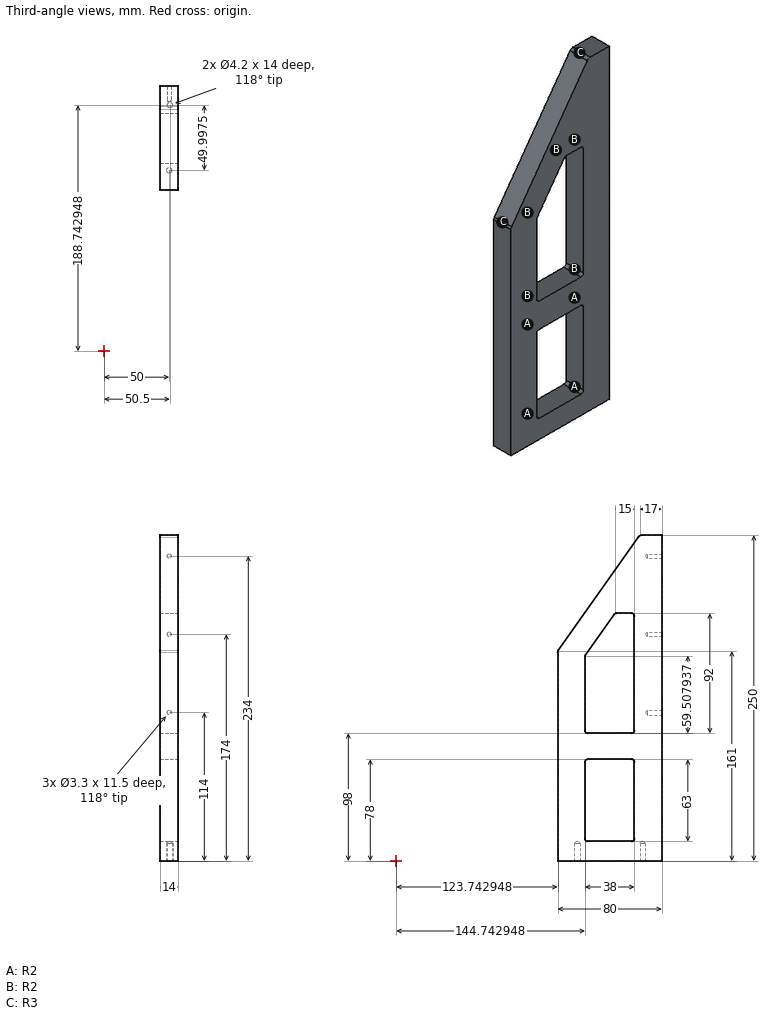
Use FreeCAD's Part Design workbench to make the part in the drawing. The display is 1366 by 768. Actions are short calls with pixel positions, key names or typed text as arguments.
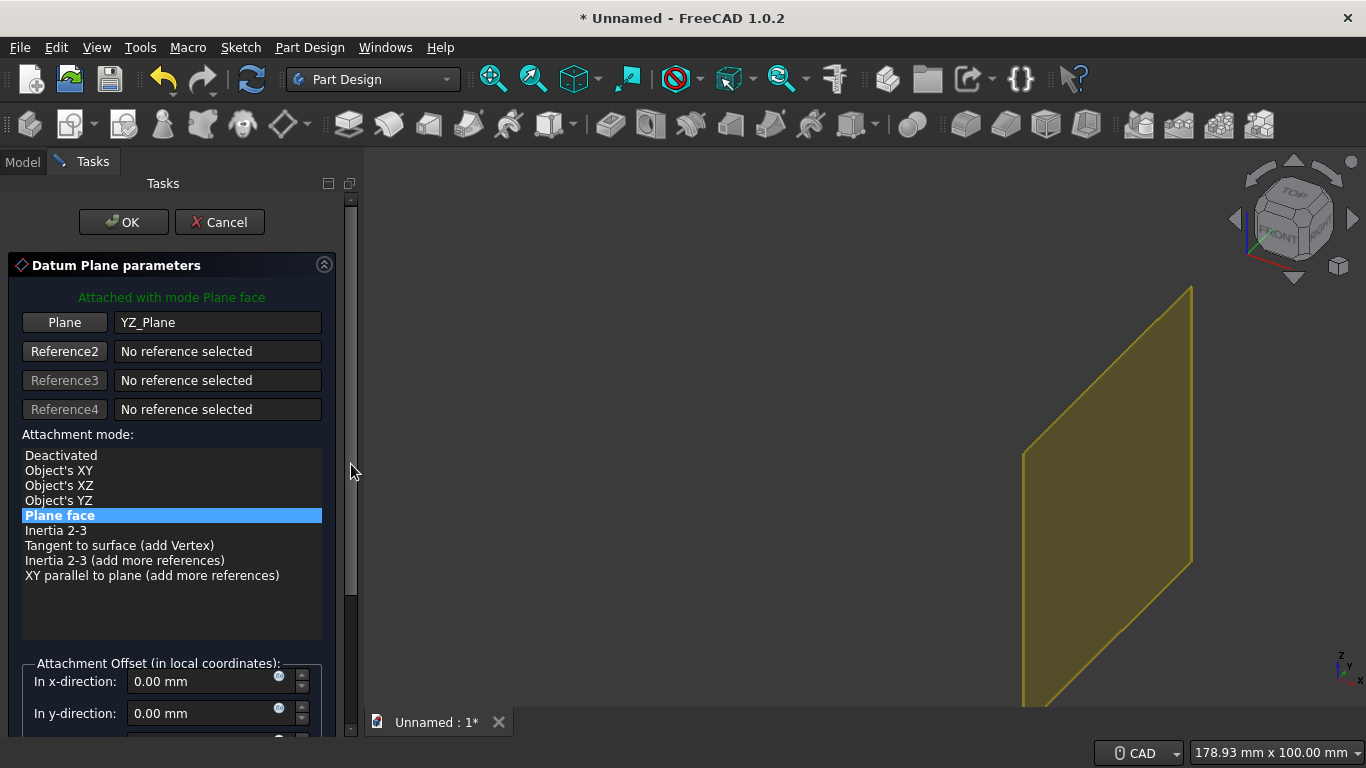
click(124, 222)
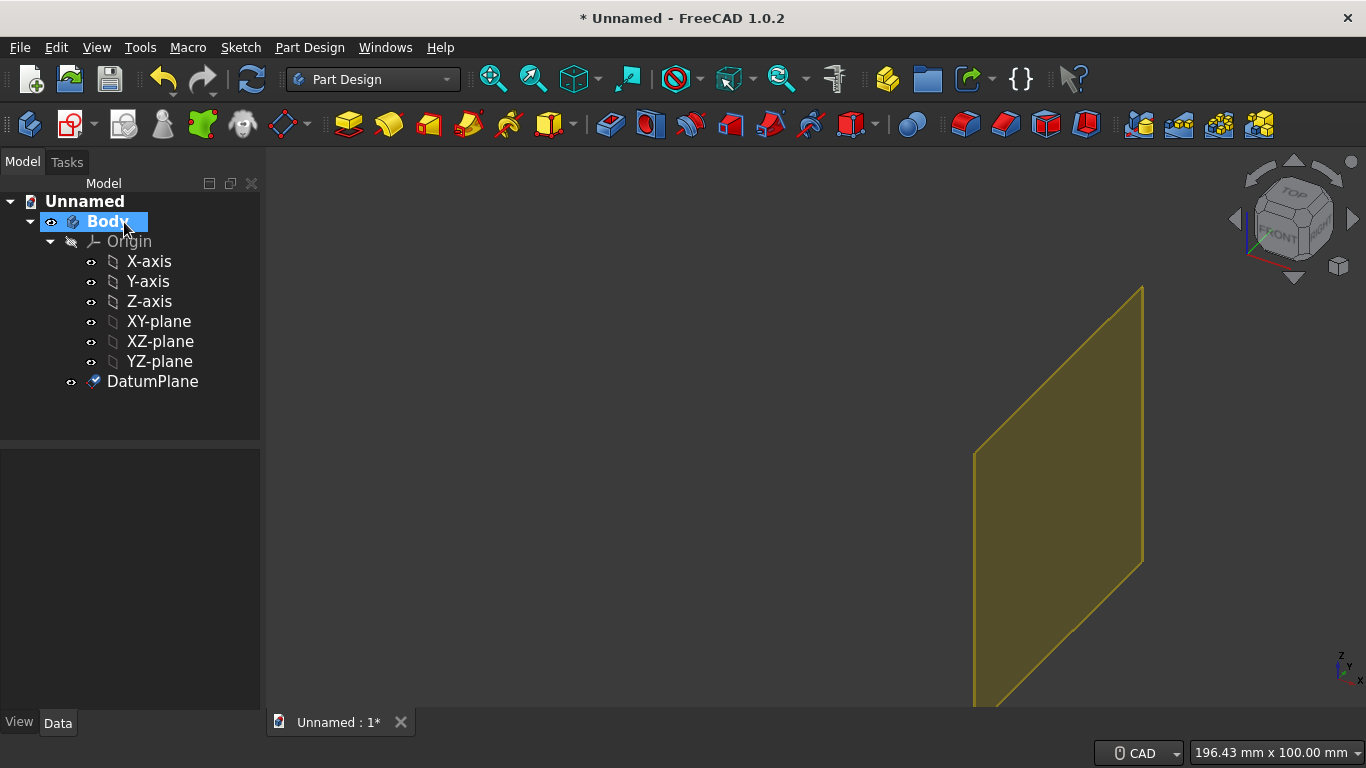
click(116, 382)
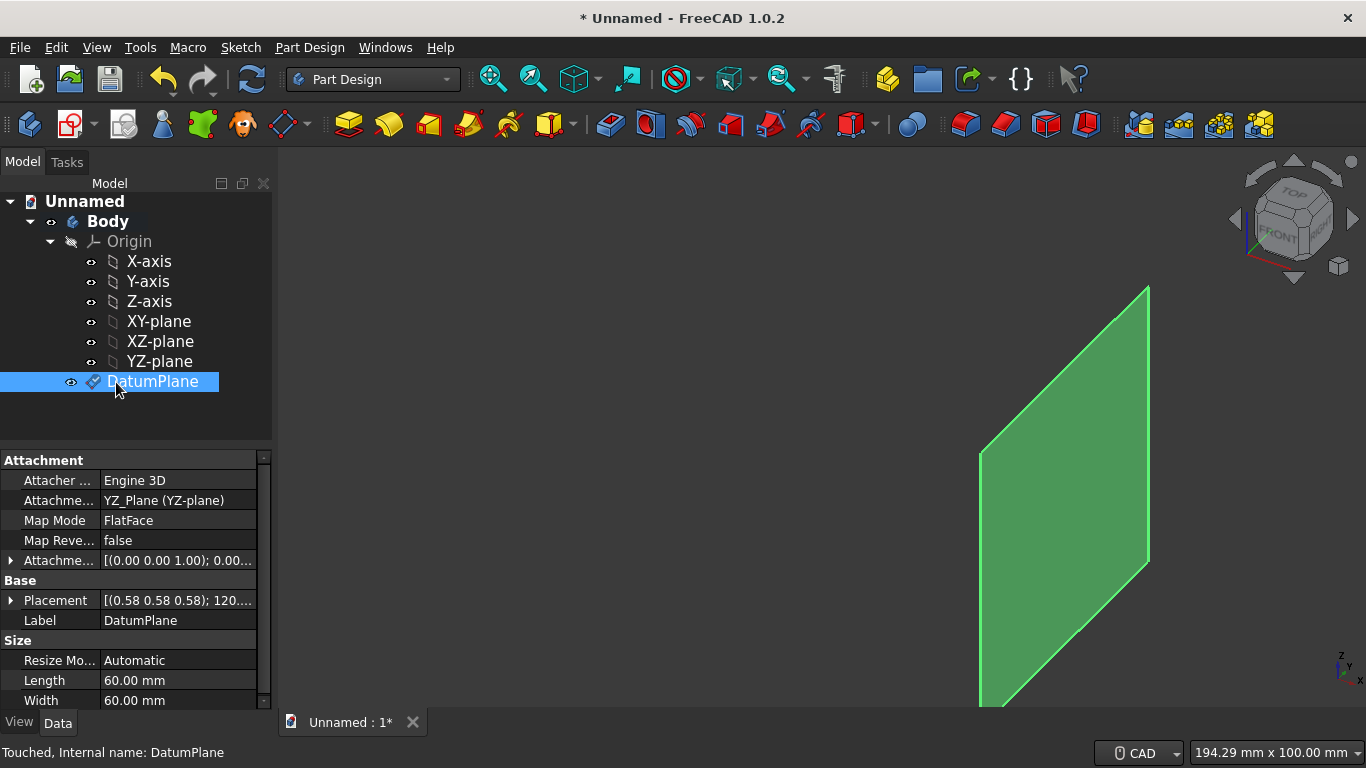
click(70, 124)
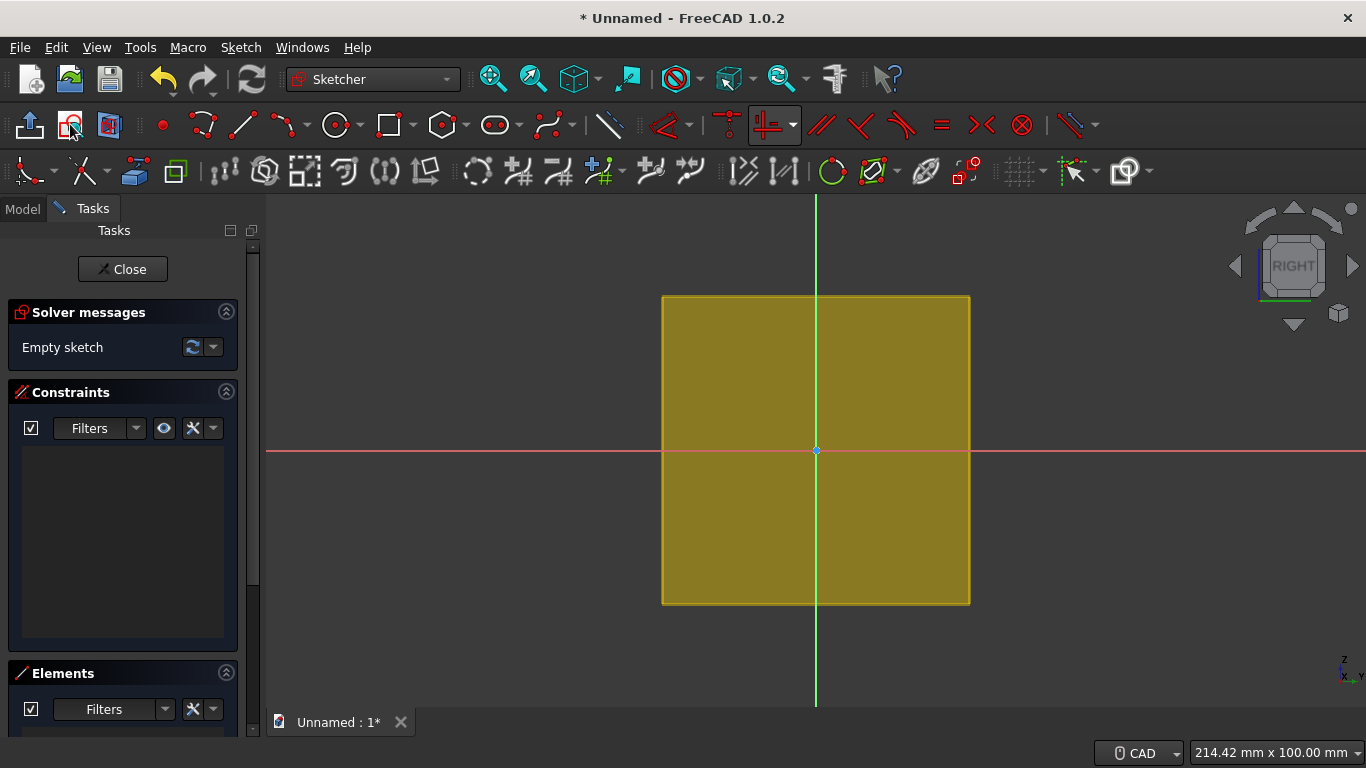
scroll(554, 660, down, 7)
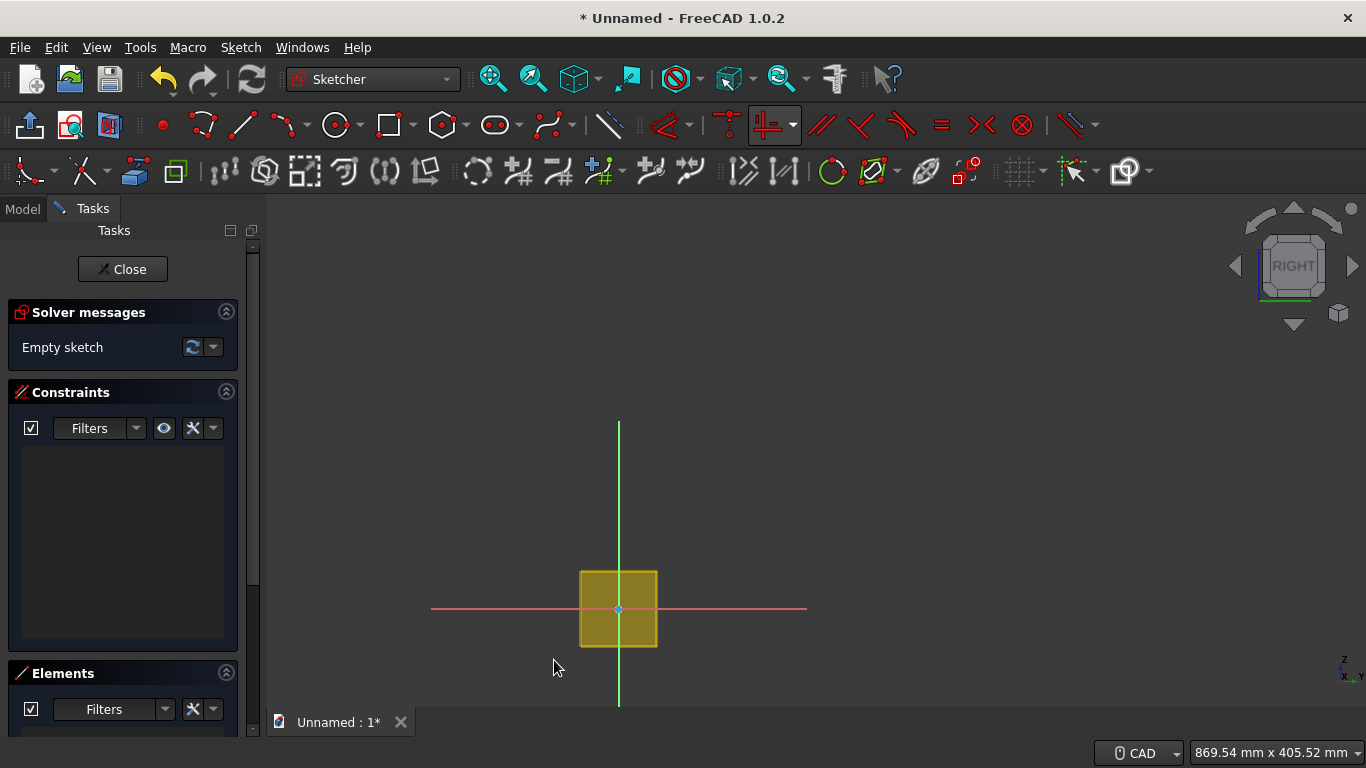
click(204, 126)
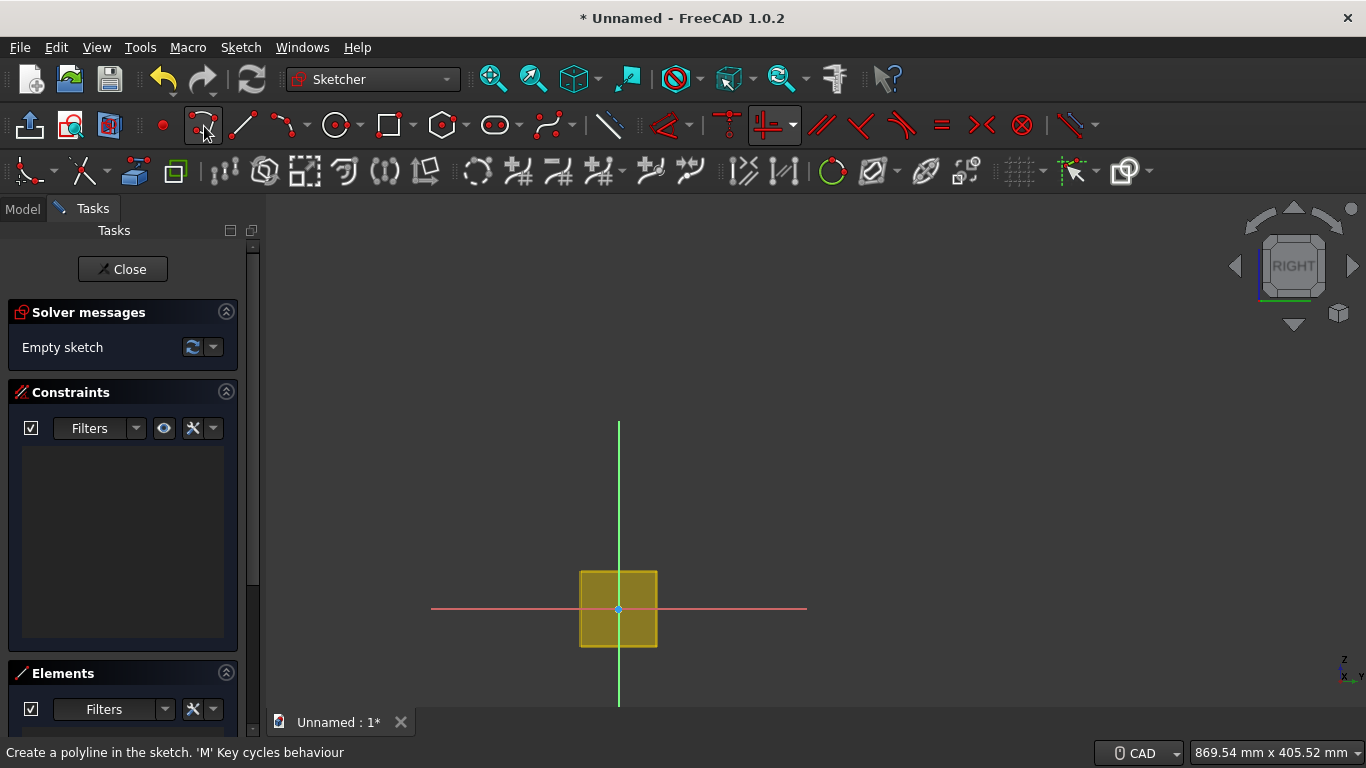
click(775, 609)
click(775, 405)
click(855, 293)
click(877, 293)
click(877, 600)
click(775, 609)
key(Escape)
key(Escape)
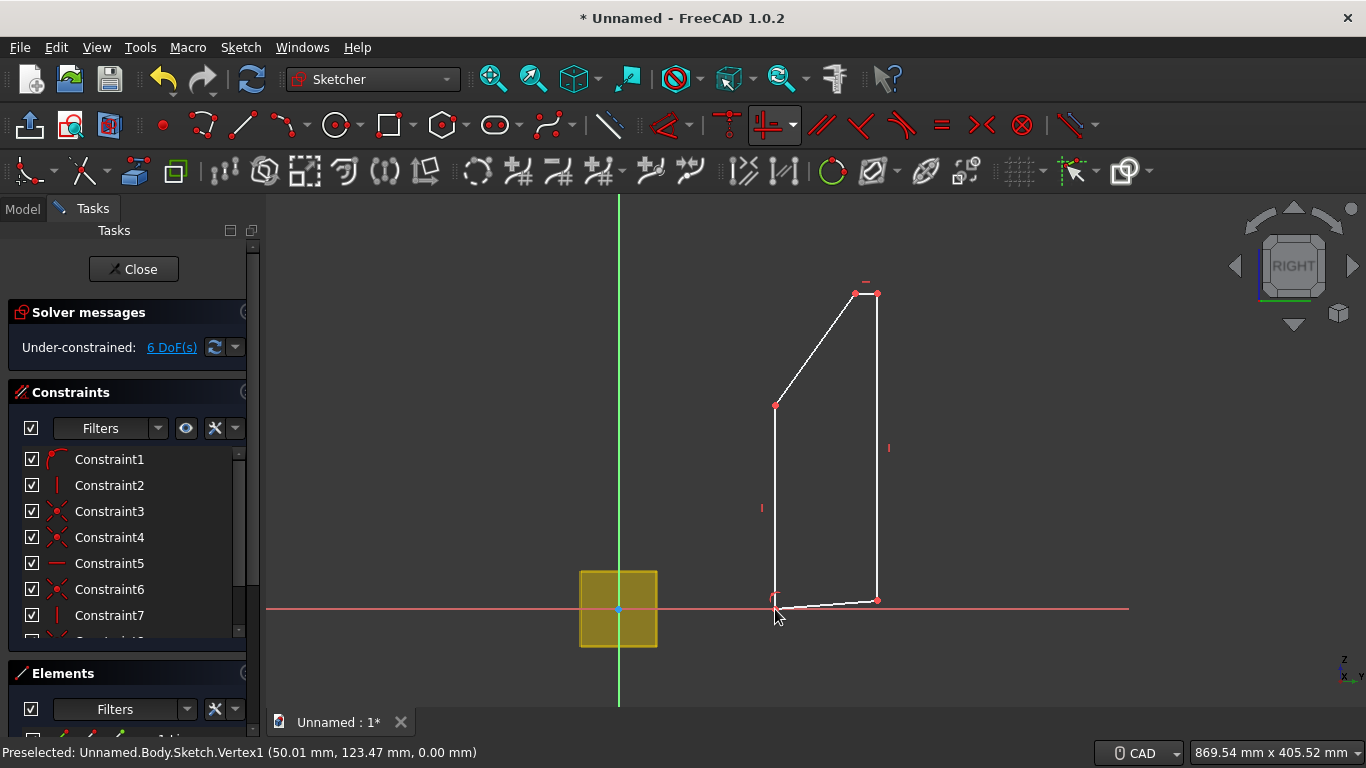
click(806, 607)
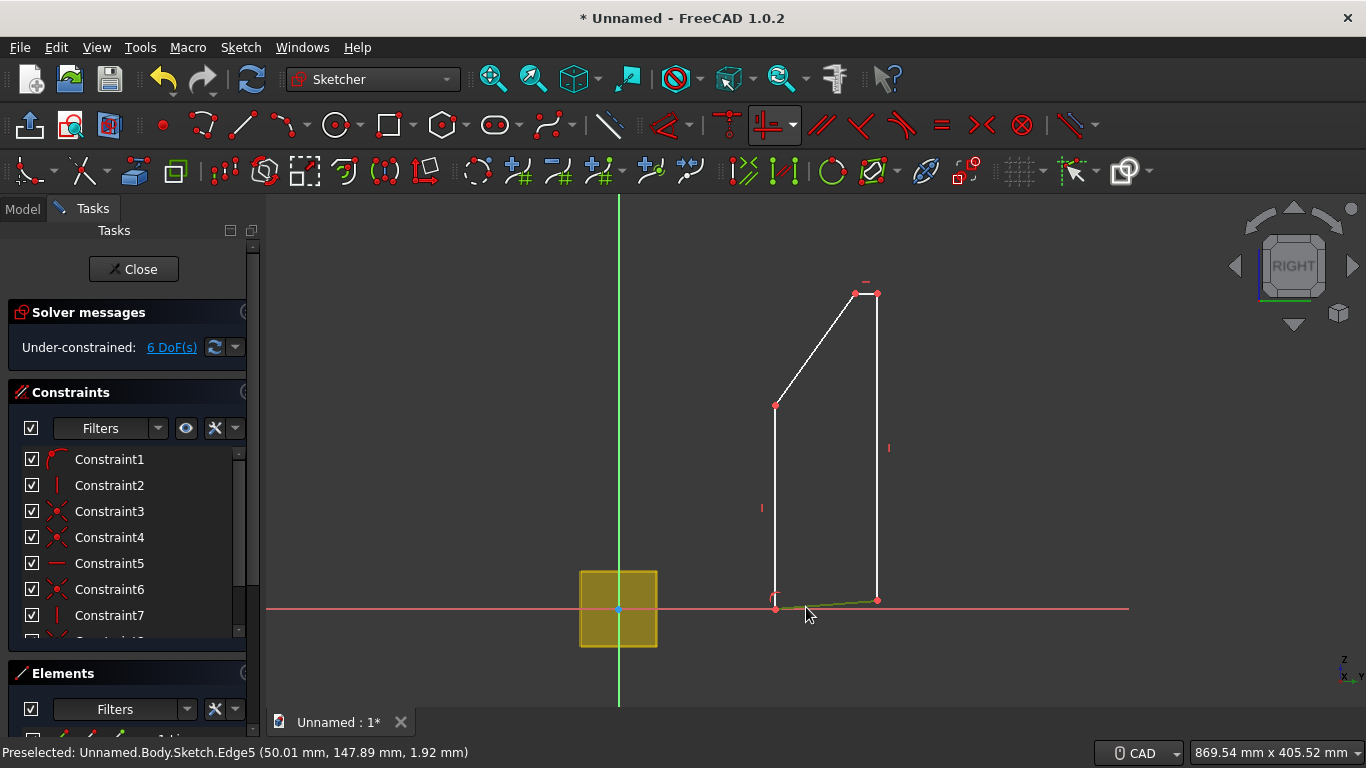
click(796, 126)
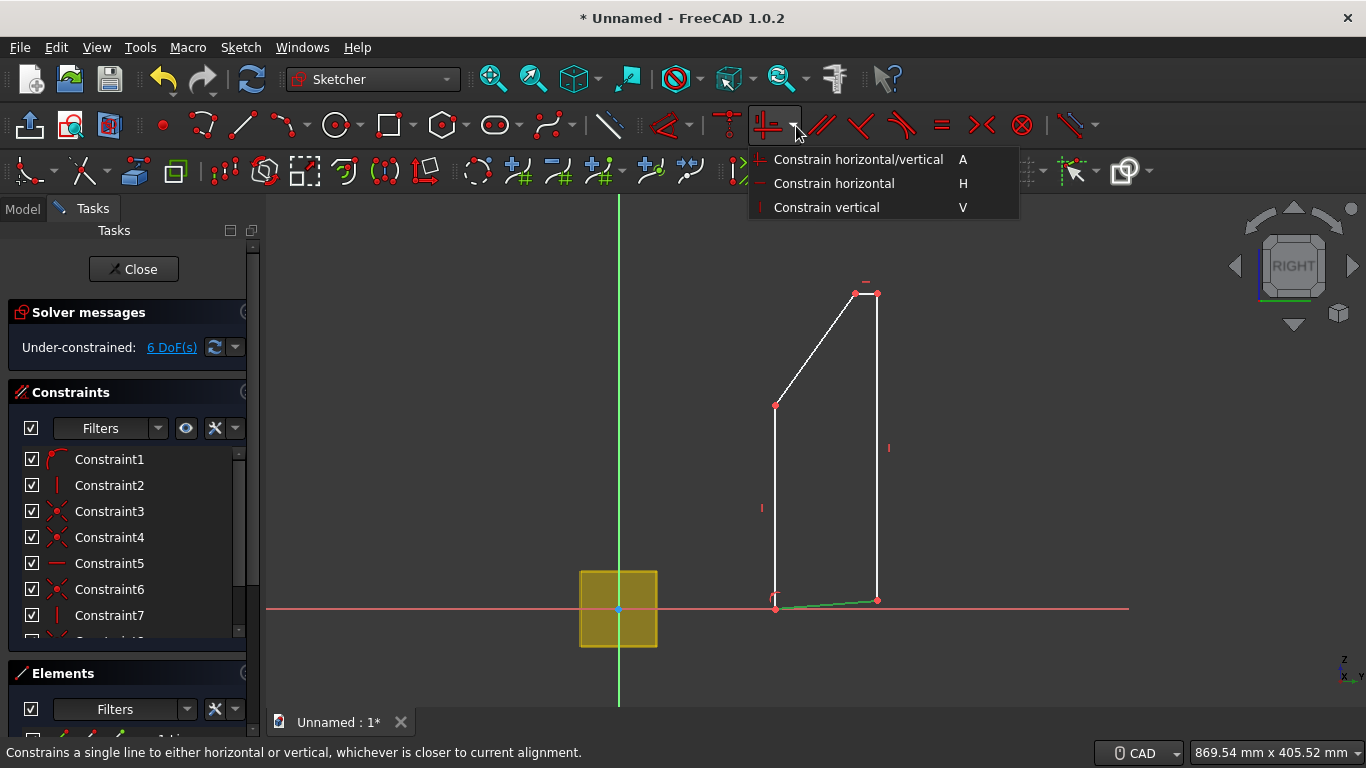
click(884, 183)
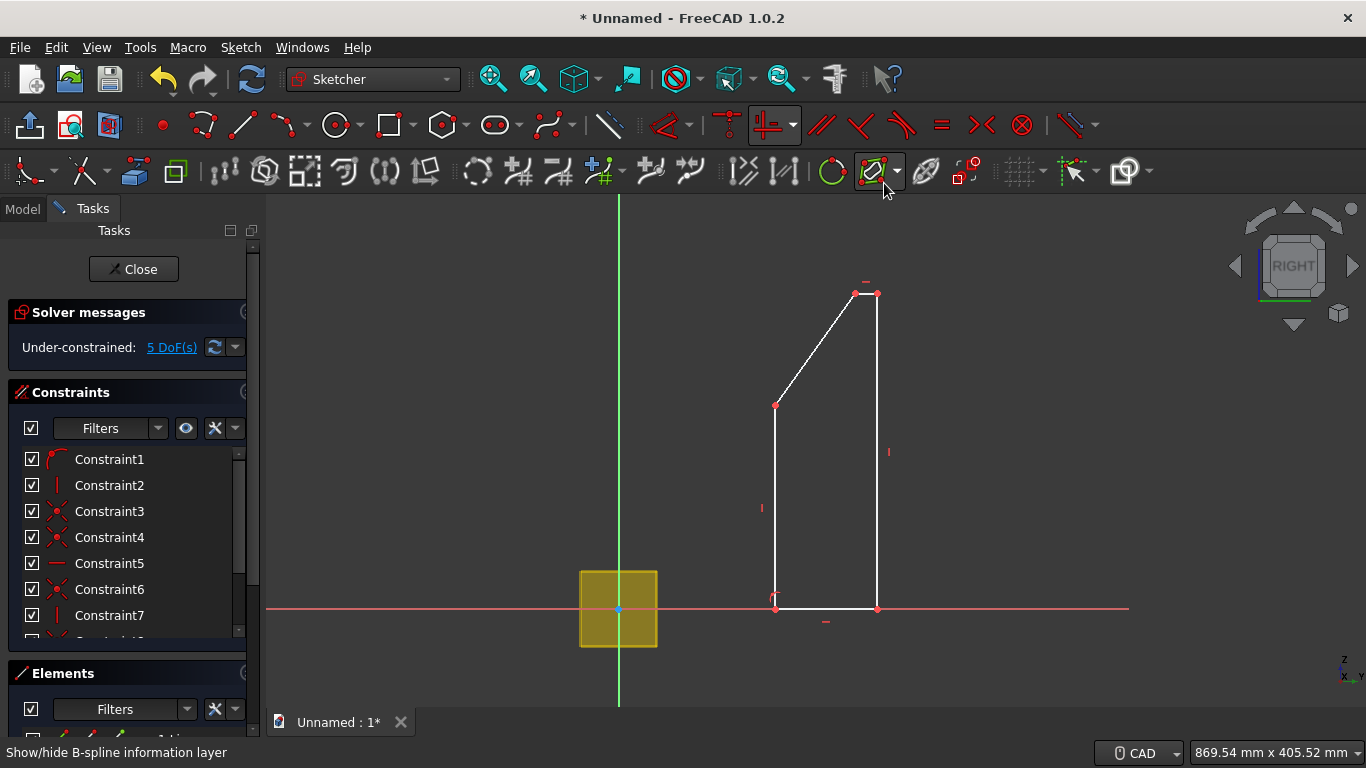
click(664, 126)